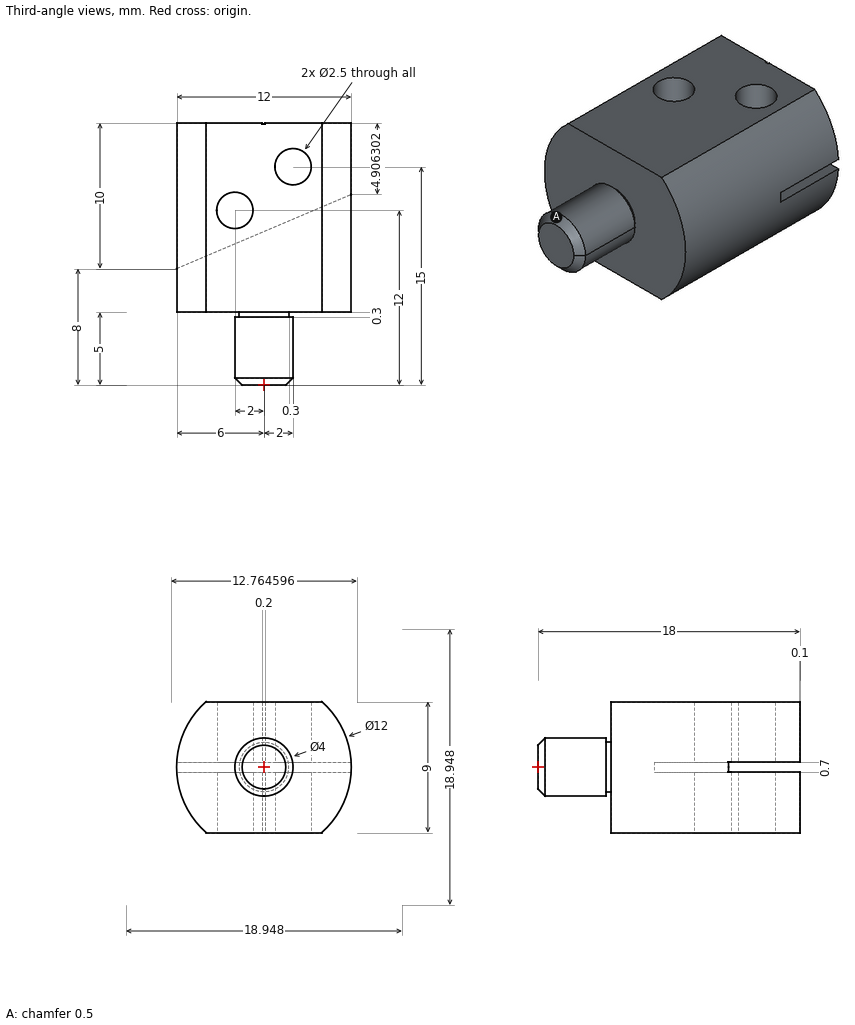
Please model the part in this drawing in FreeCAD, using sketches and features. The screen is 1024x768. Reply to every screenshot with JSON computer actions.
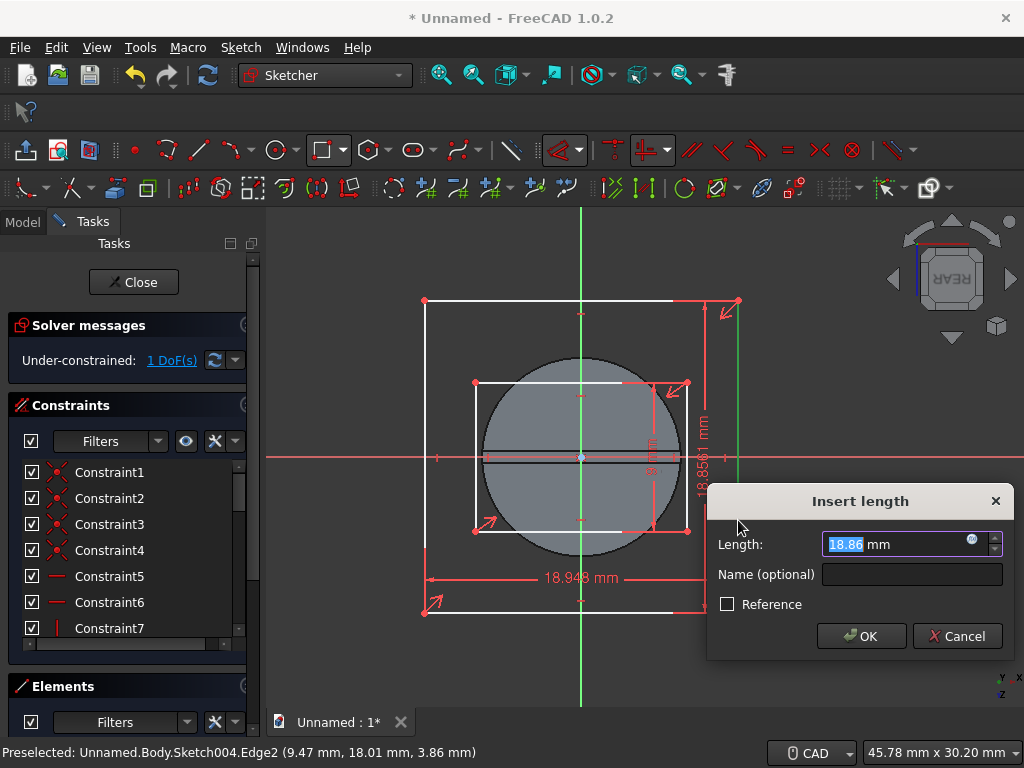
{"action": "type", "text": "18.948"}
{"action": "key", "text": "Return"}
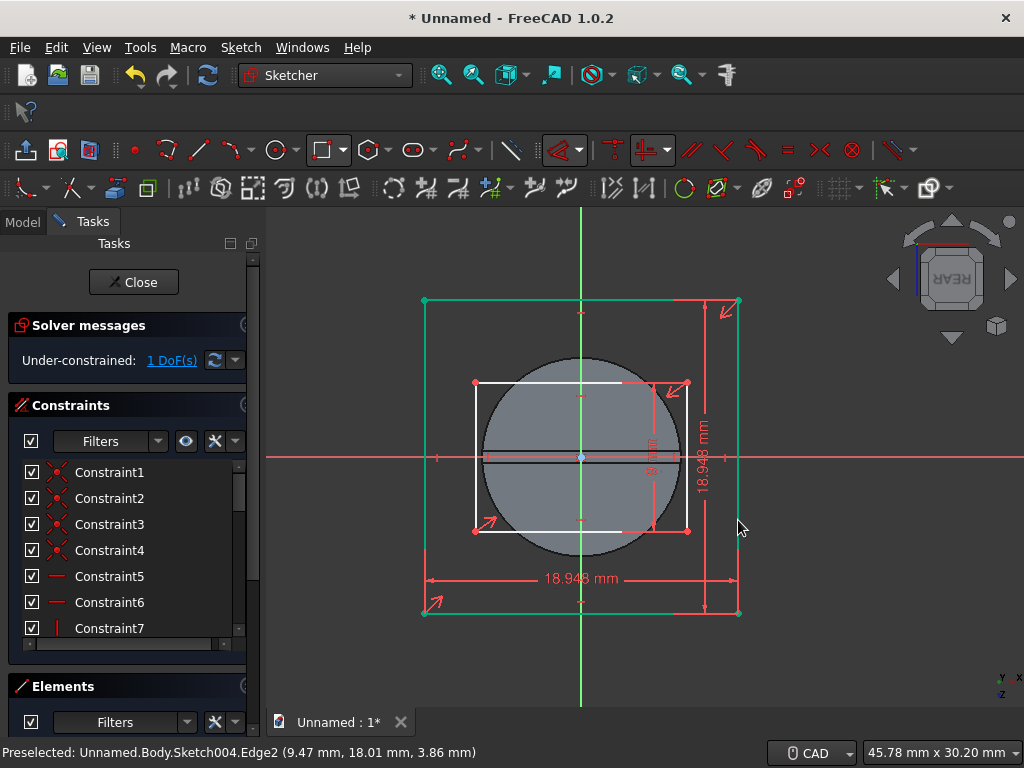
{"action": "left_click", "coordinate": [539, 532]}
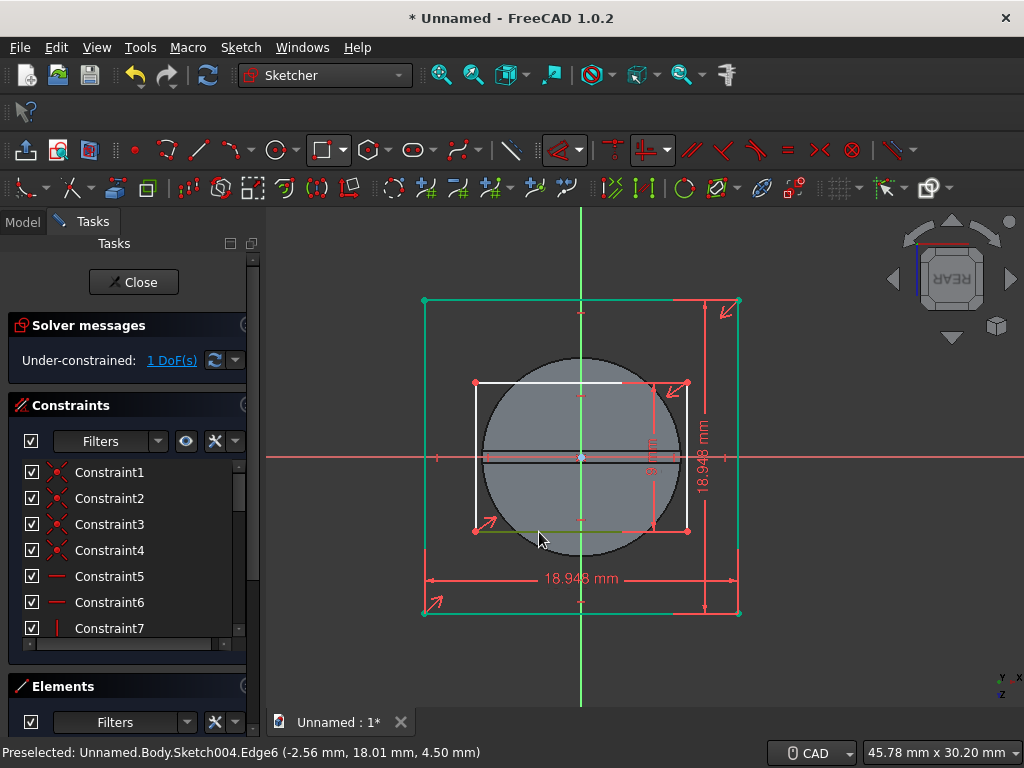
{"action": "key", "text": "l"}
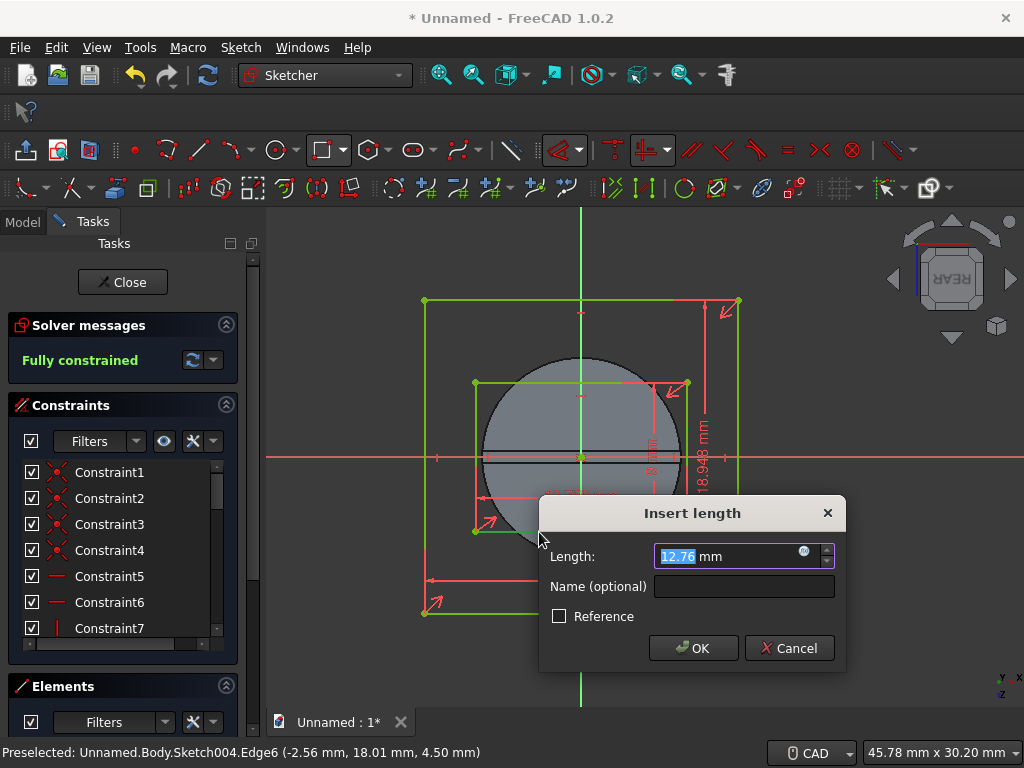
{"action": "type", "text": "12.764596"}
{"action": "key", "text": "Return"}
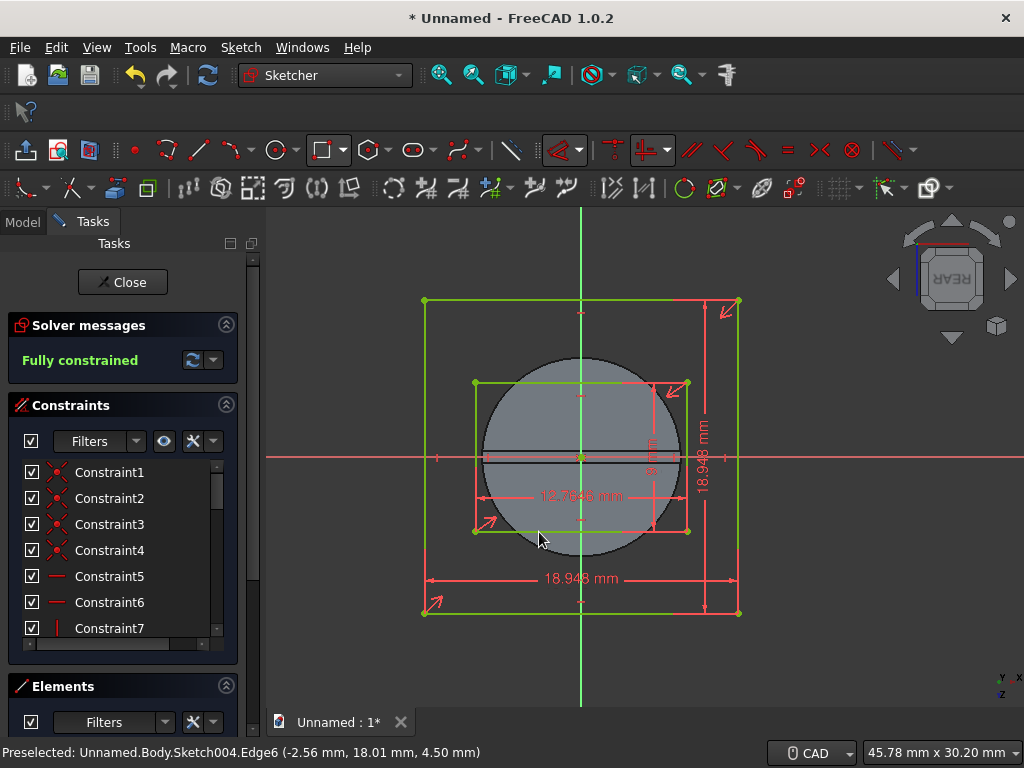
{"action": "left_click", "coordinate": [123, 282]}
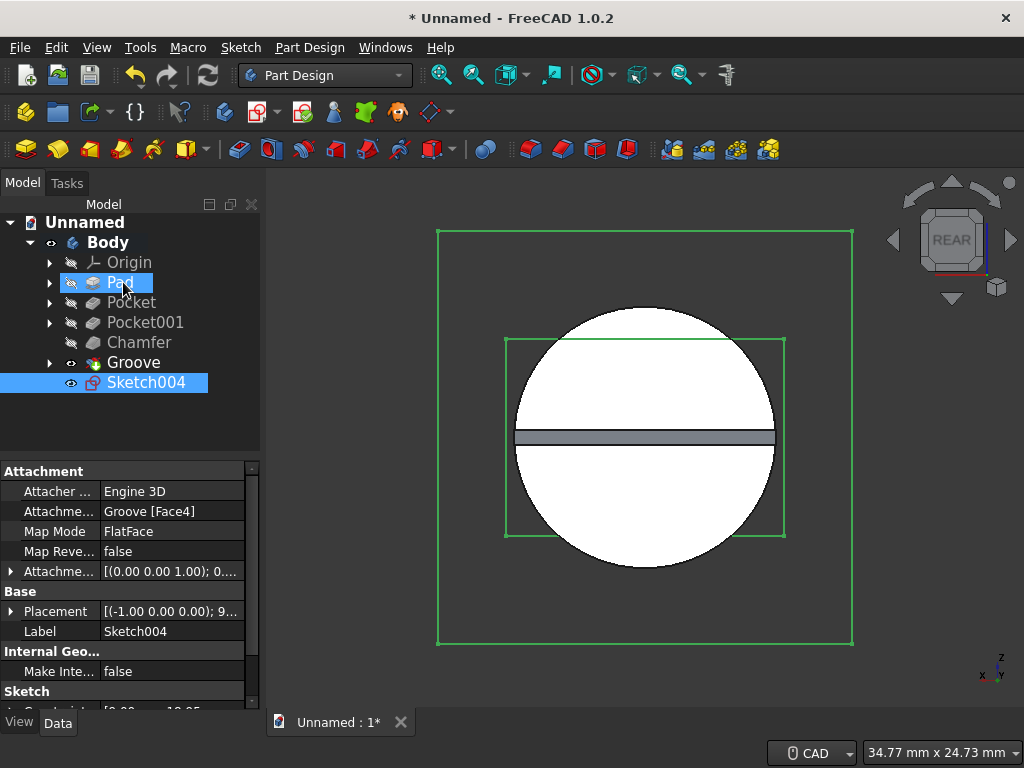
{"action": "left_click", "coordinate": [240, 150]}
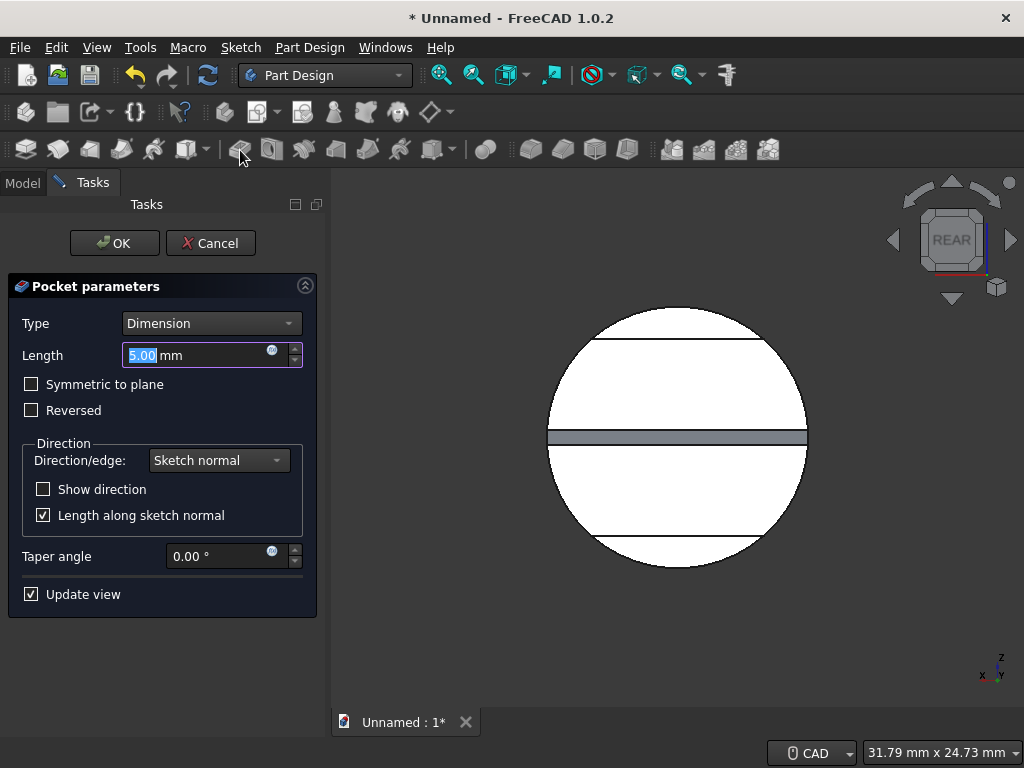
{"action": "left_click", "coordinate": [212, 324]}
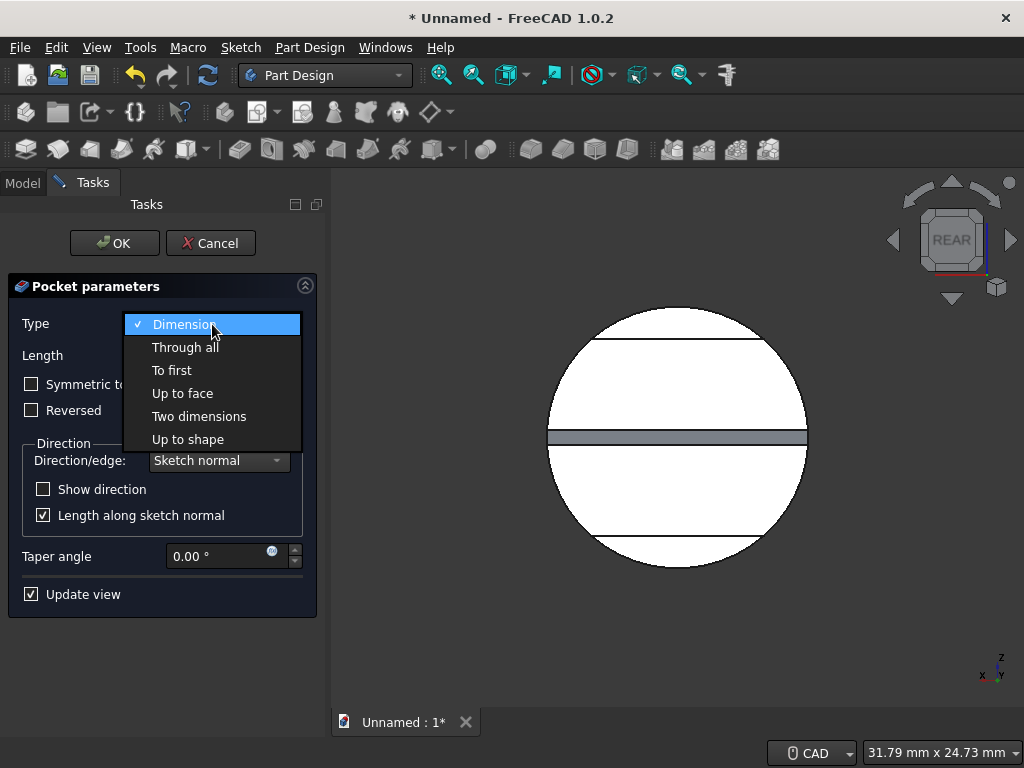
{"action": "left_click", "coordinate": [212, 348]}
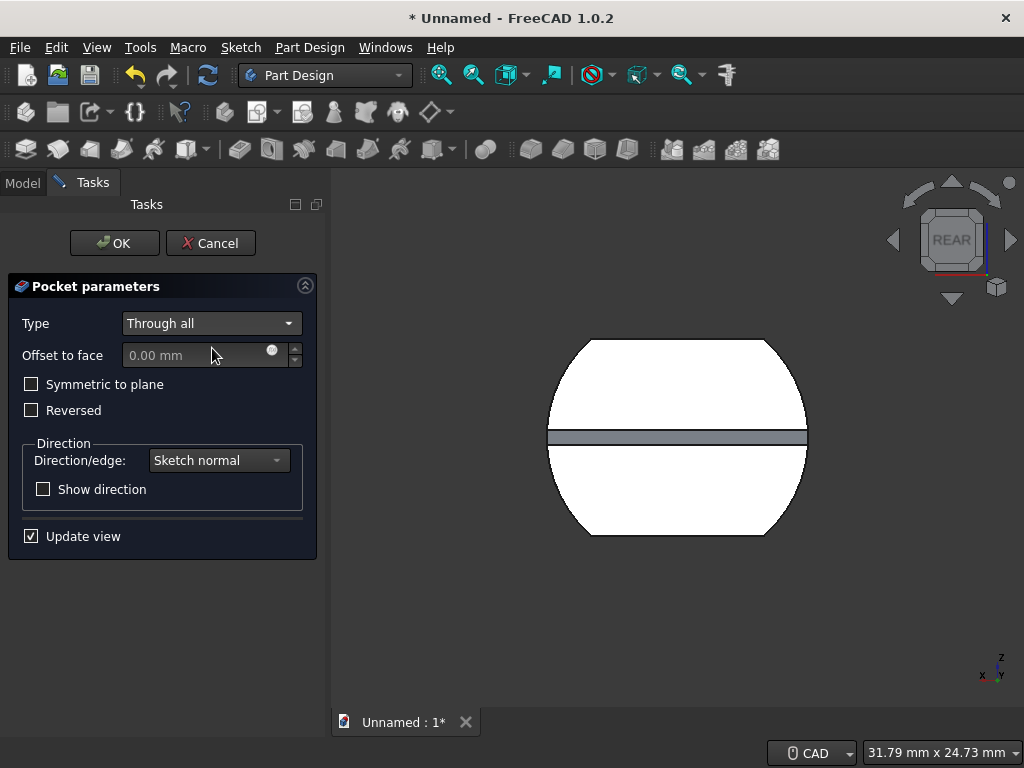
{"action": "left_click", "coordinate": [115, 243]}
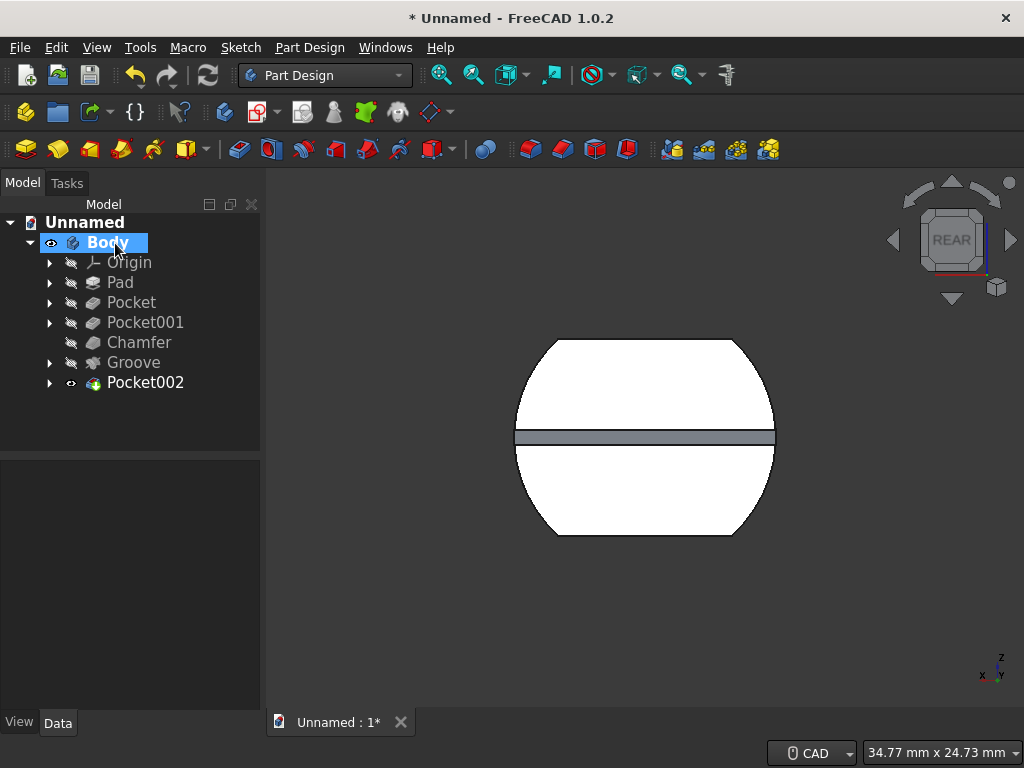
{"action": "left_click", "coordinate": [442, 76]}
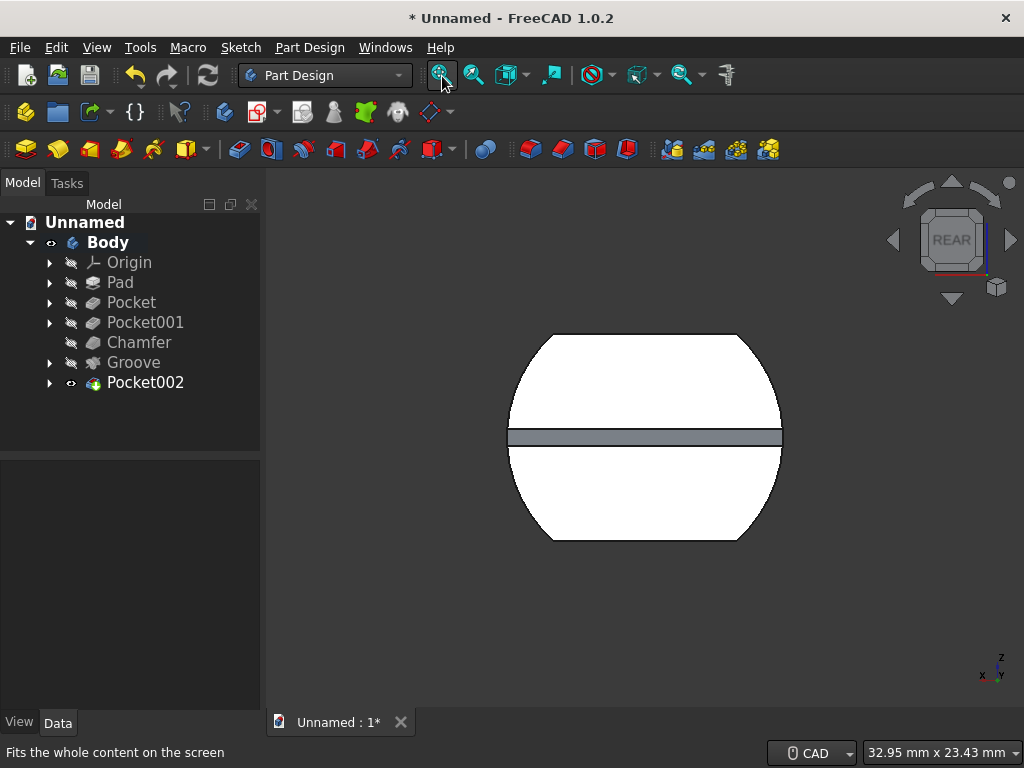
{"action": "key", "text": "0"}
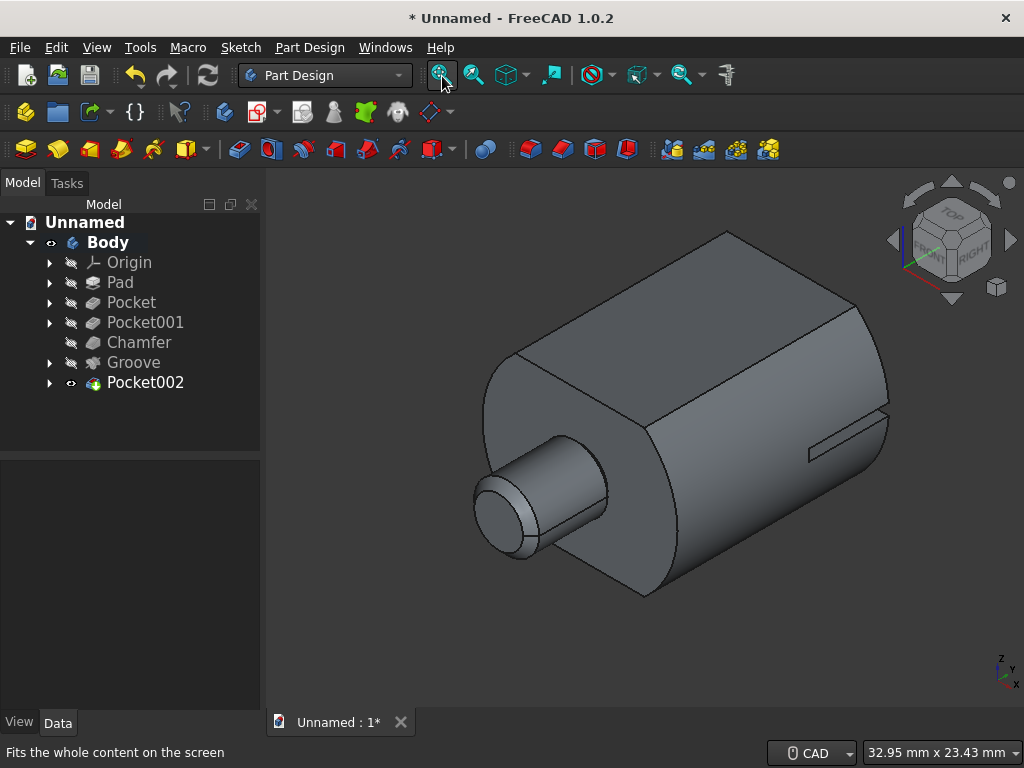
{"action": "left_click", "coordinate": [716, 311]}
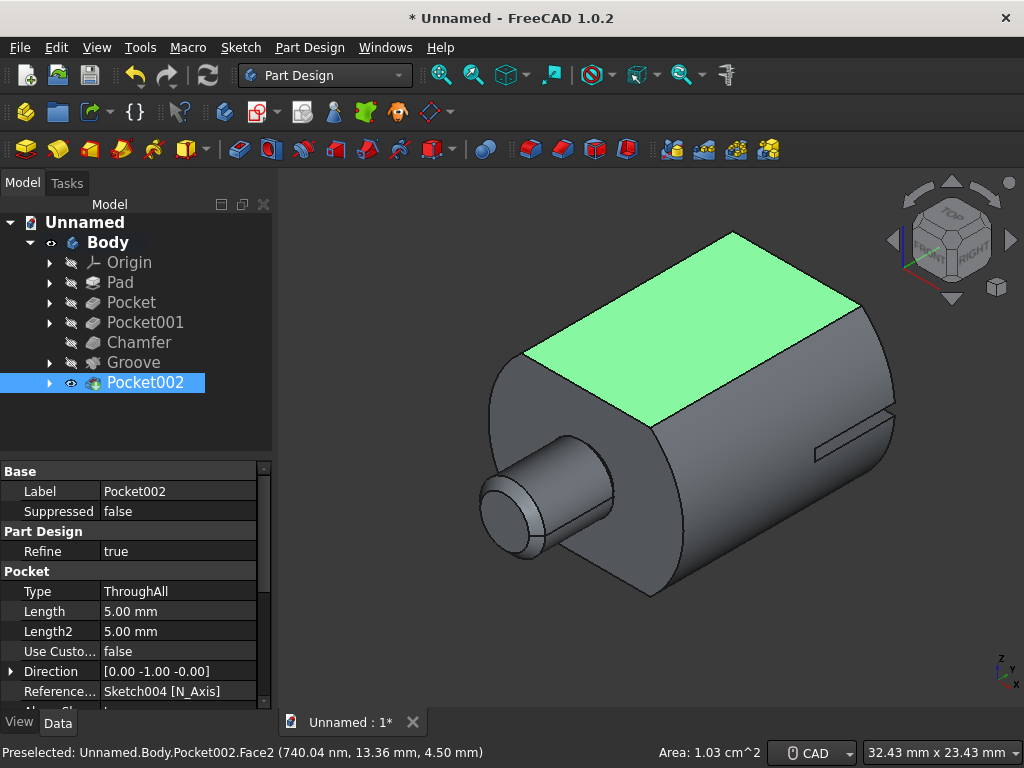
{"action": "left_click", "coordinate": [258, 112]}